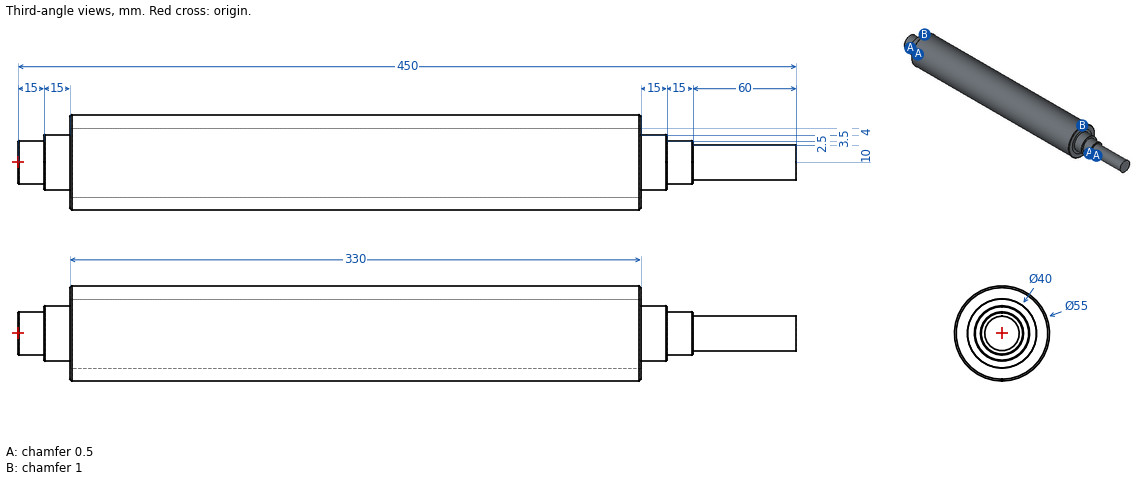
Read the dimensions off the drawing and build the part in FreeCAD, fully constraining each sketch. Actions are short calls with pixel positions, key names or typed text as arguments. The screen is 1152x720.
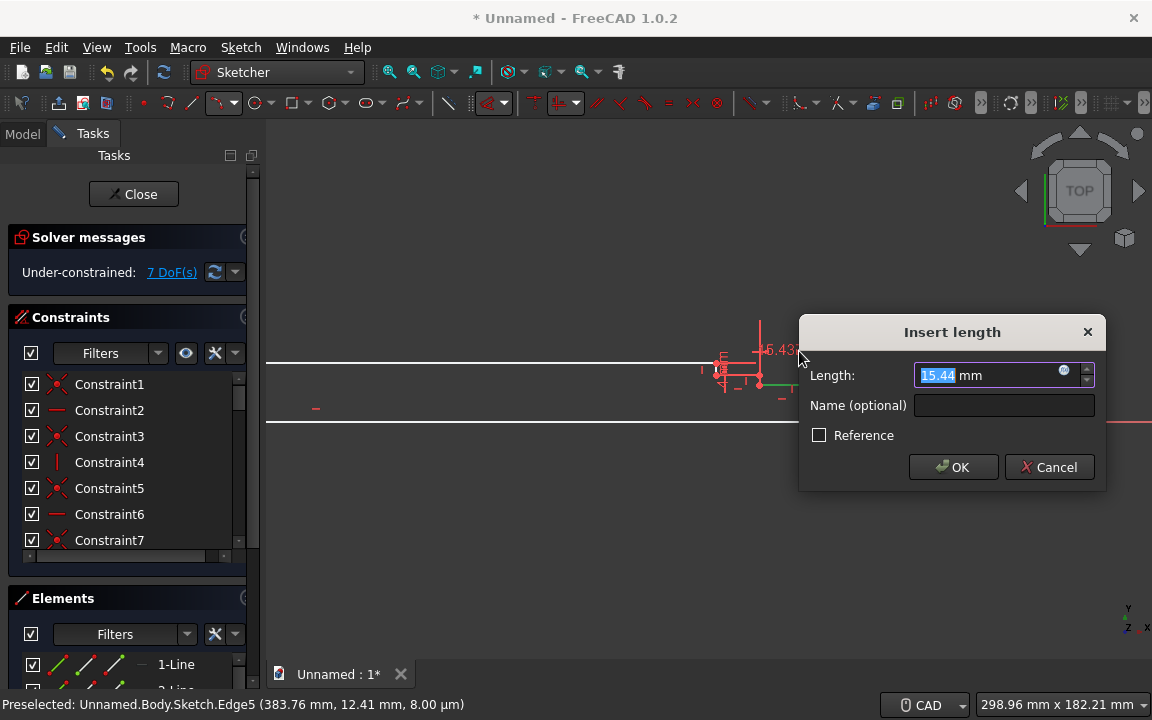
text(15)
key(Return)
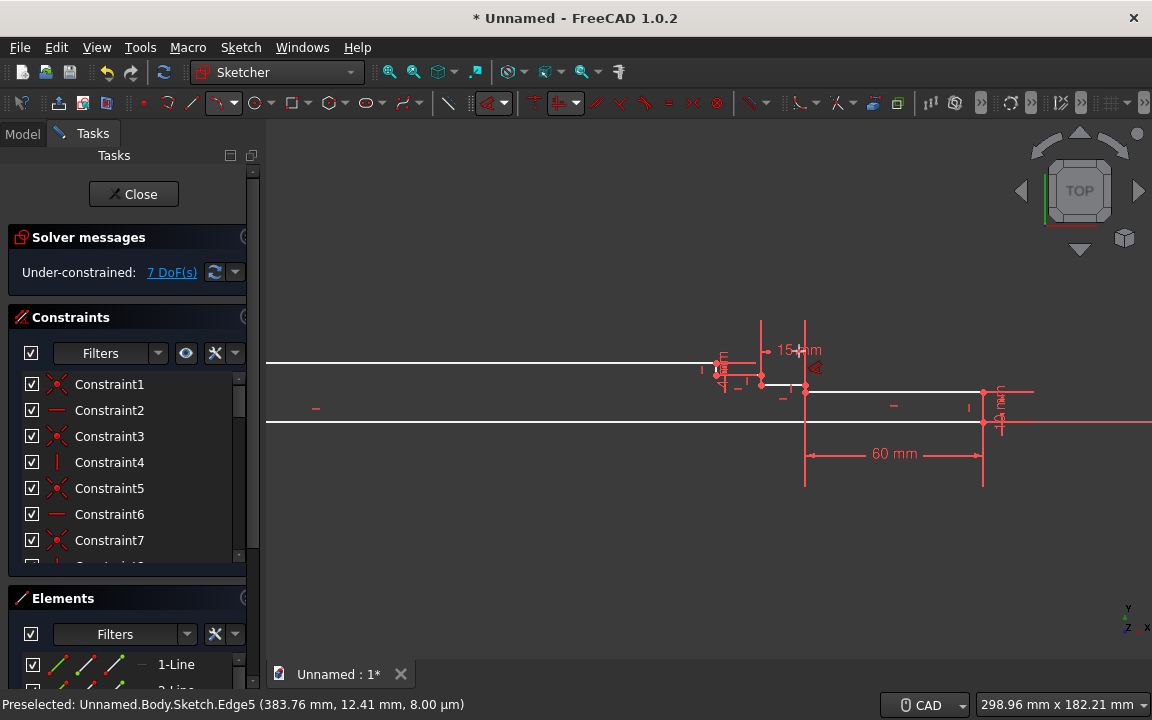
click(748, 375)
click(728, 341)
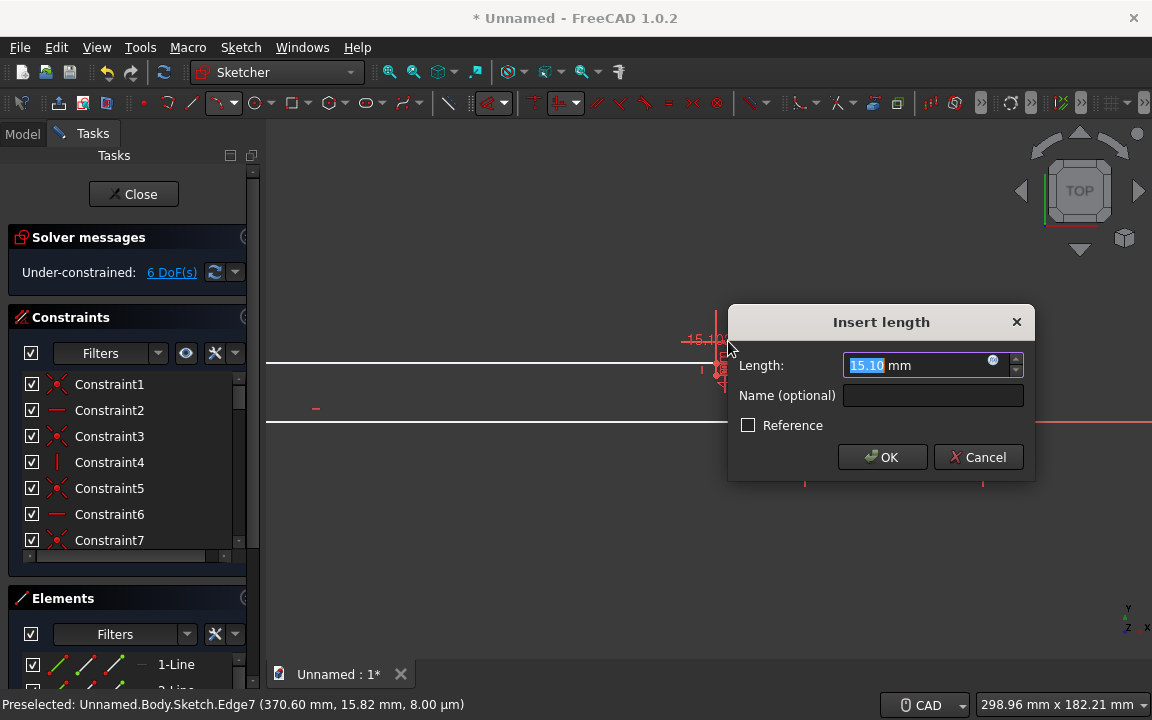
text(15)
key(Return)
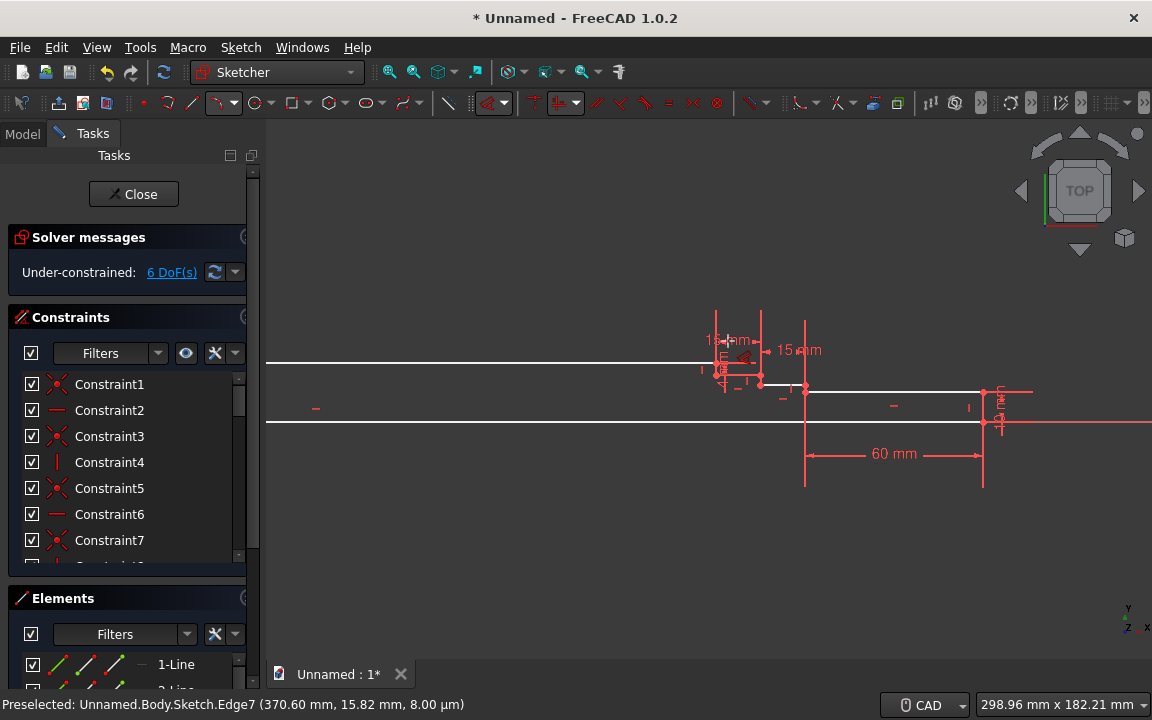
scroll(829, 387, down, 5)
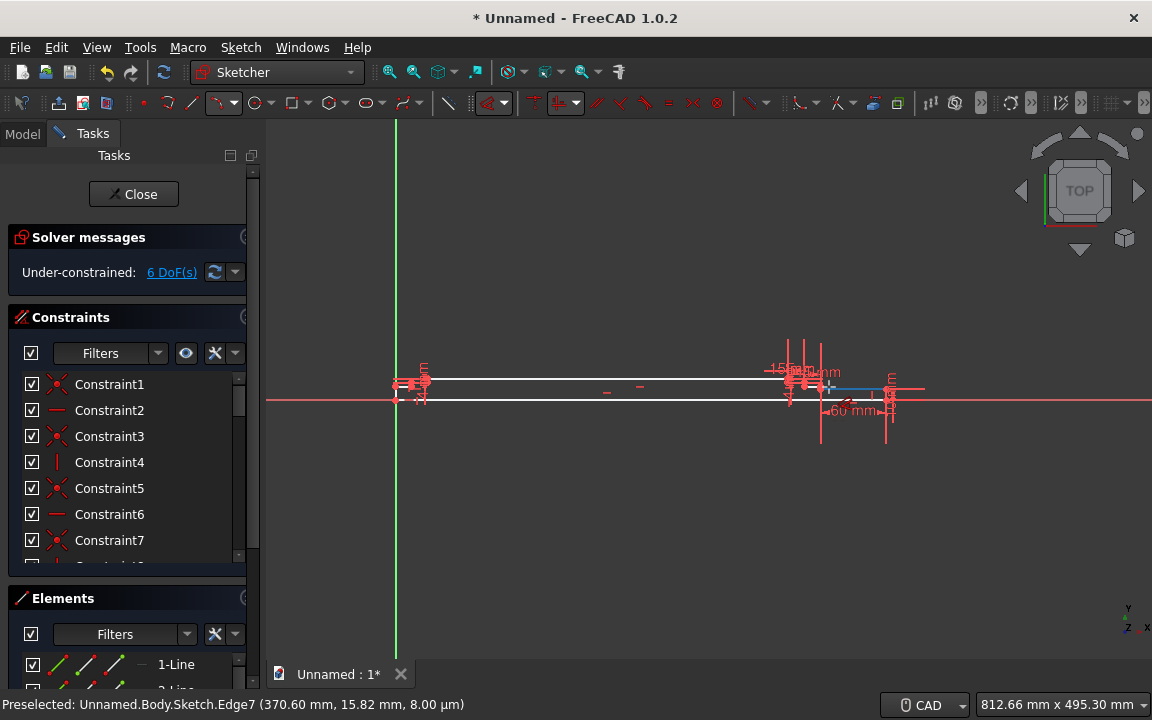
scroll(423, 383, up, 6)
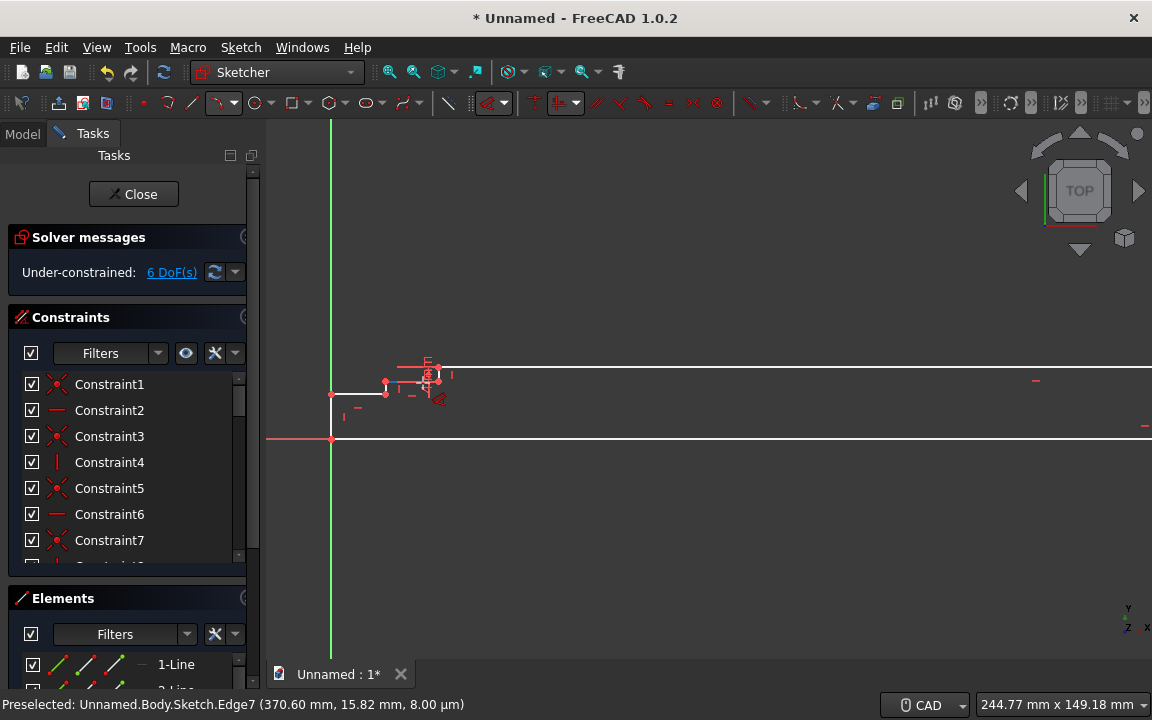
click(423, 382)
click(412, 348)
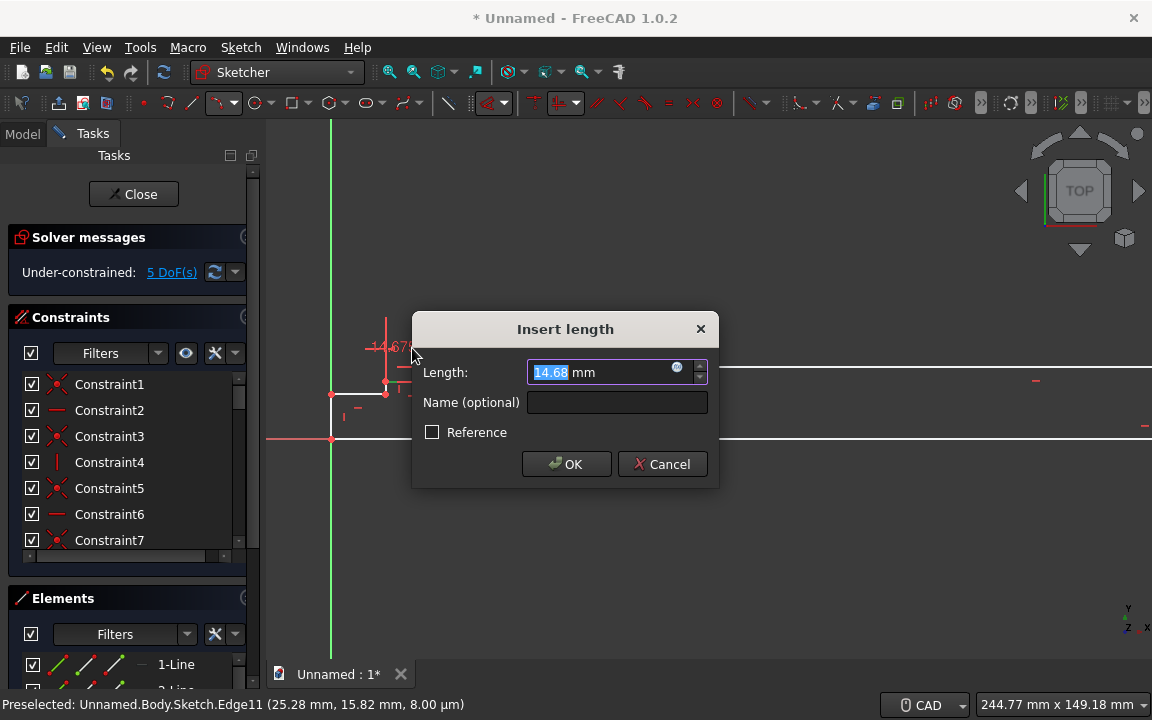
text(15)
key(Return)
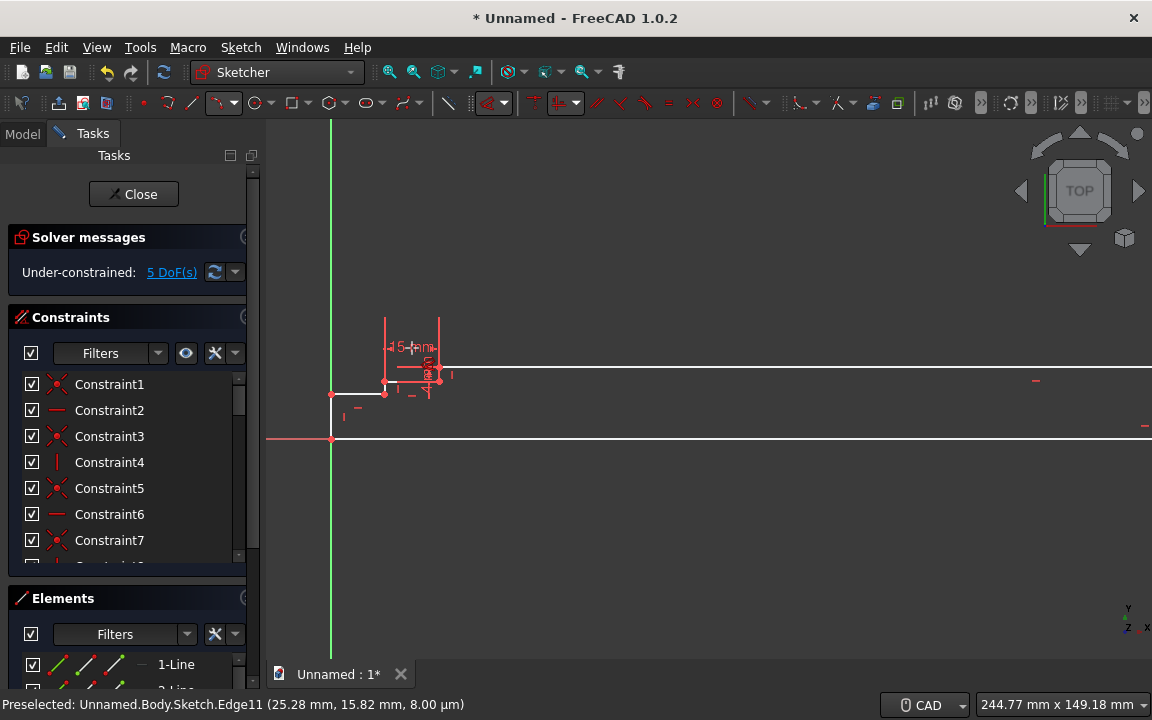
click(369, 394)
click(358, 452)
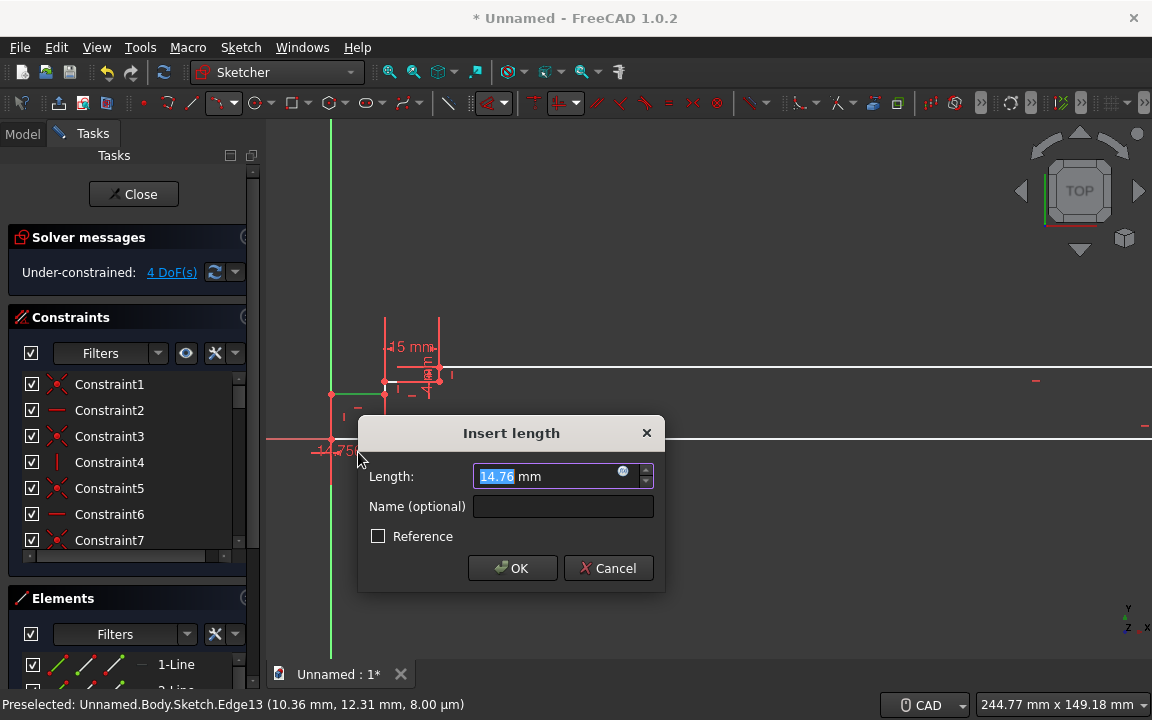
text(15)
key(Return)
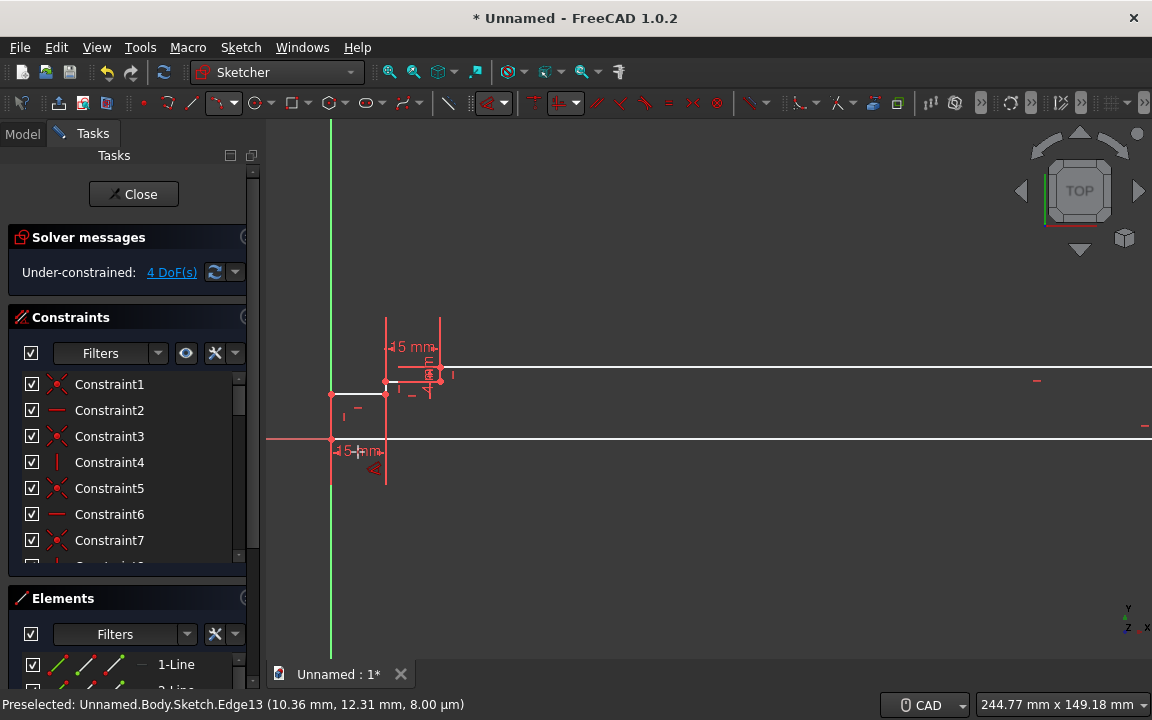
click(820, 439)
click(659, 473)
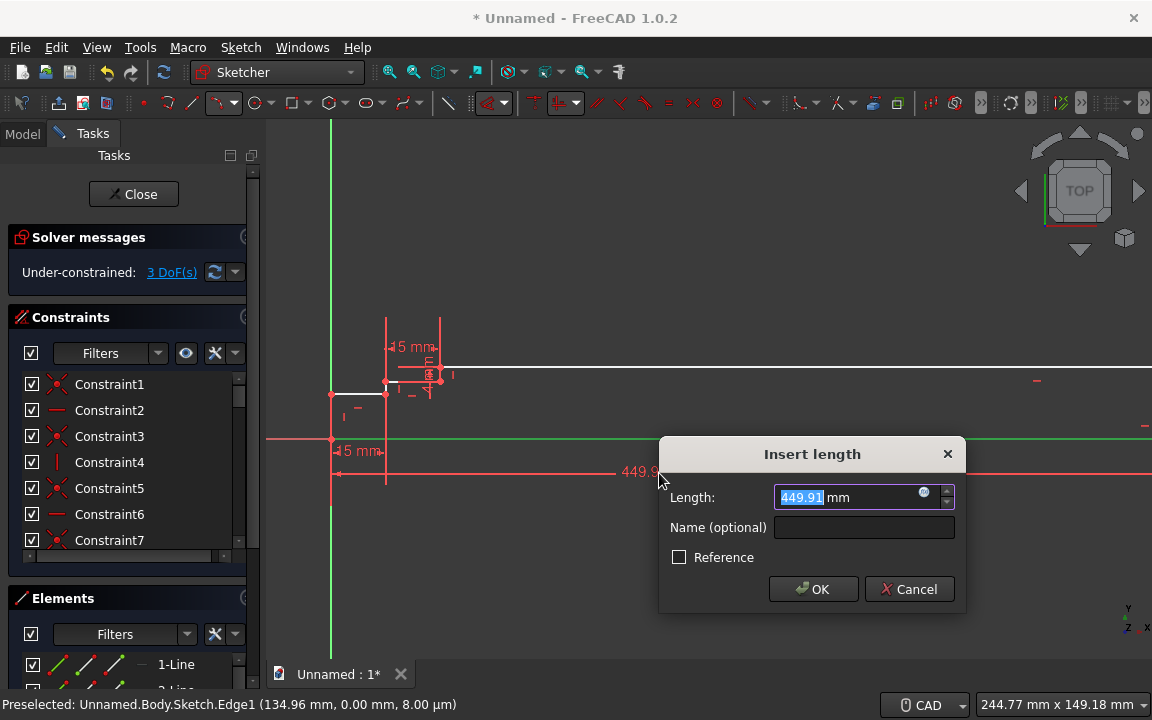
text(450)
key(Return)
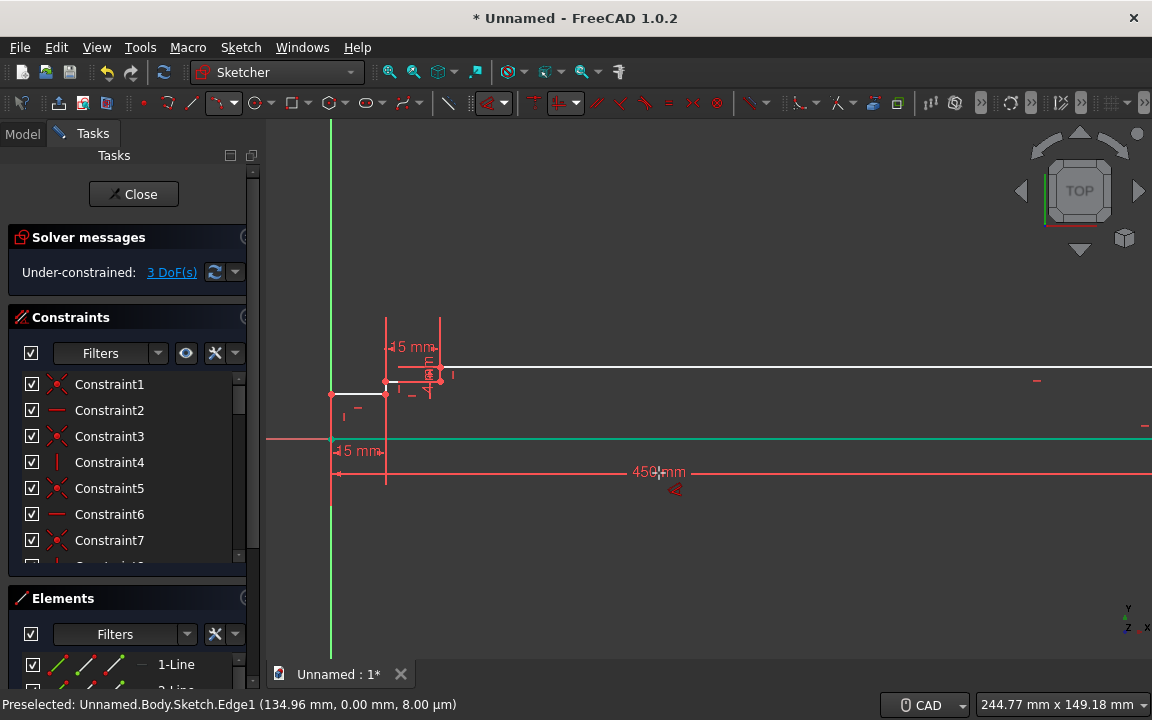
scroll(423, 383, down, 6)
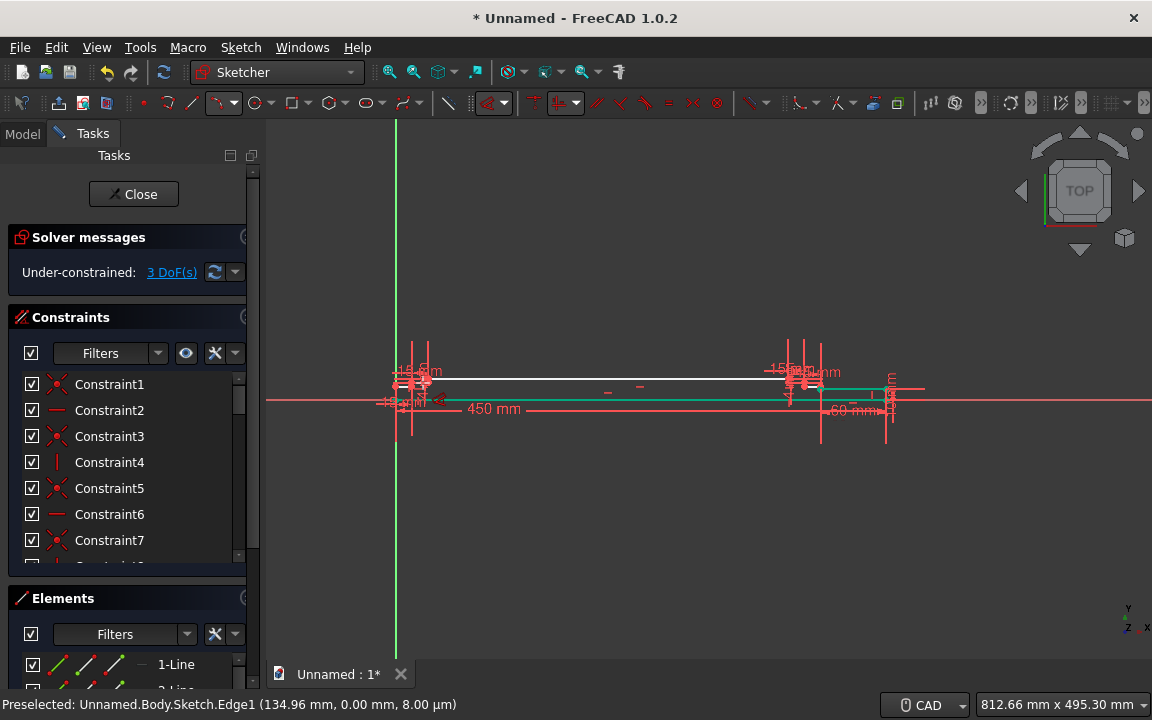
scroll(821, 388, up, 14)